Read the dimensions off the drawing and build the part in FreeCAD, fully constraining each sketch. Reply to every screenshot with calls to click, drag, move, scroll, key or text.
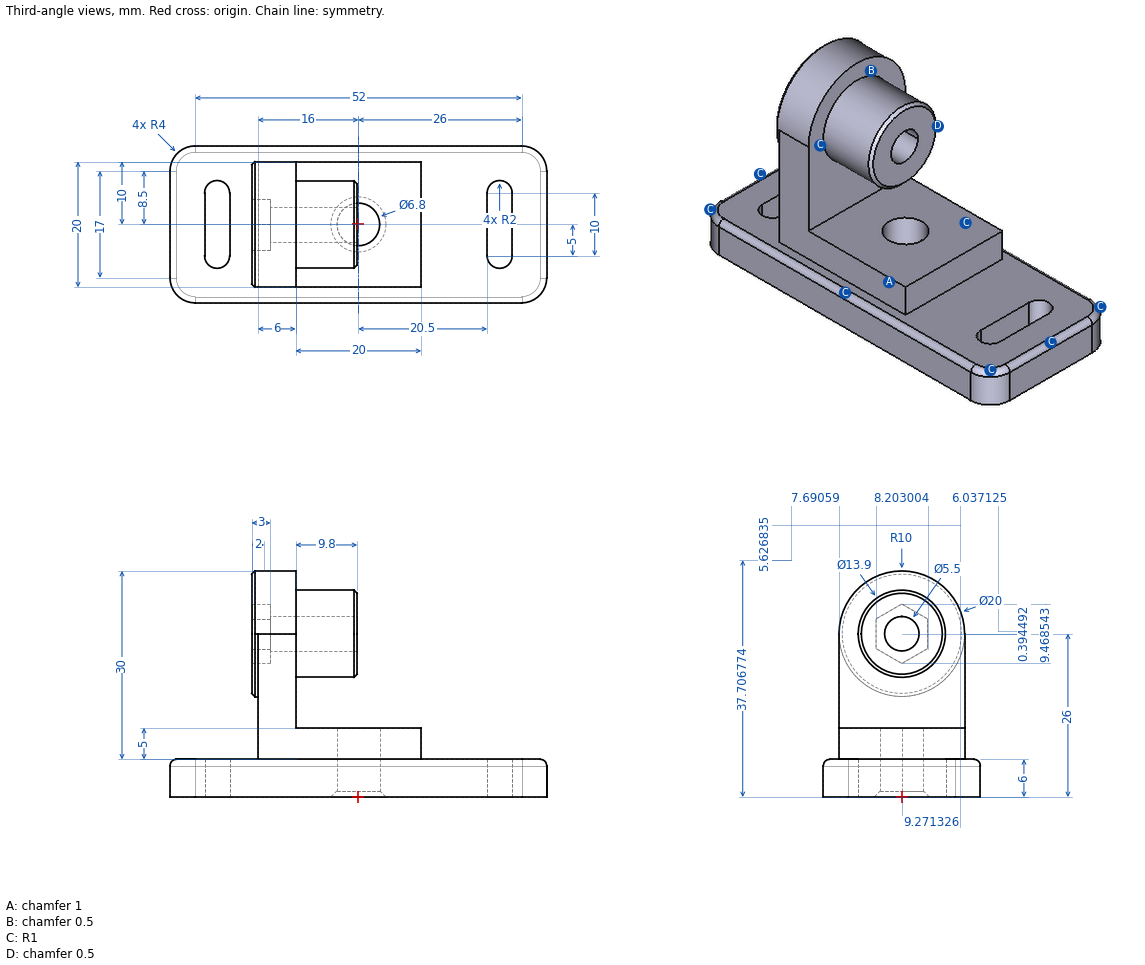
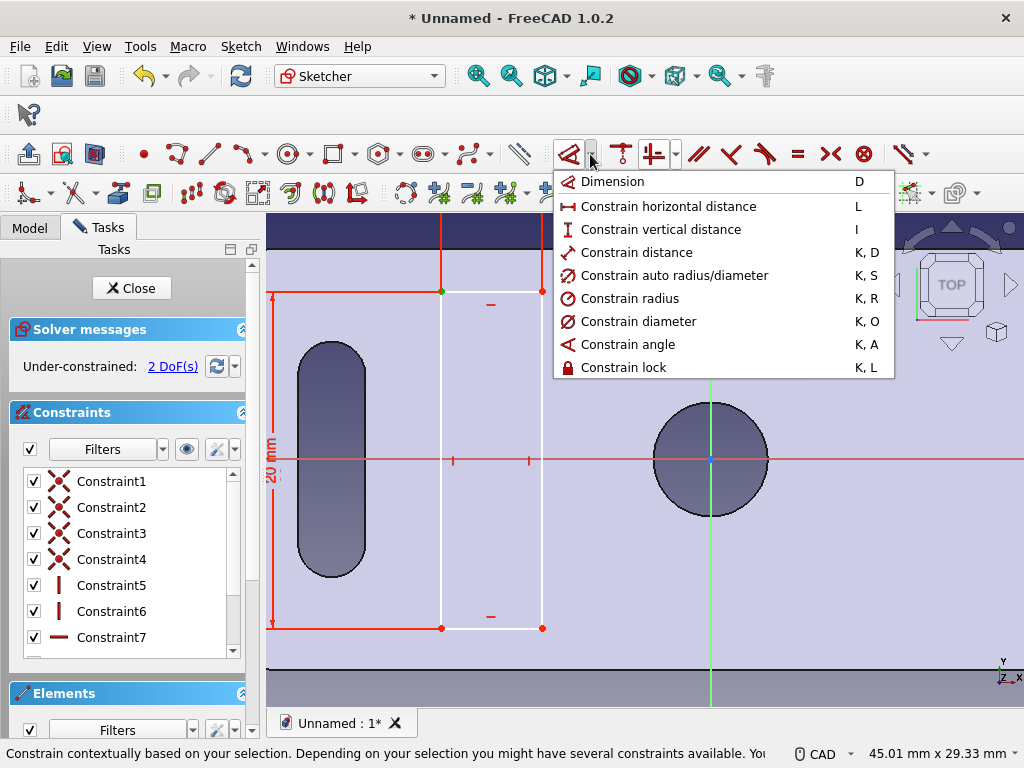
click(724, 206)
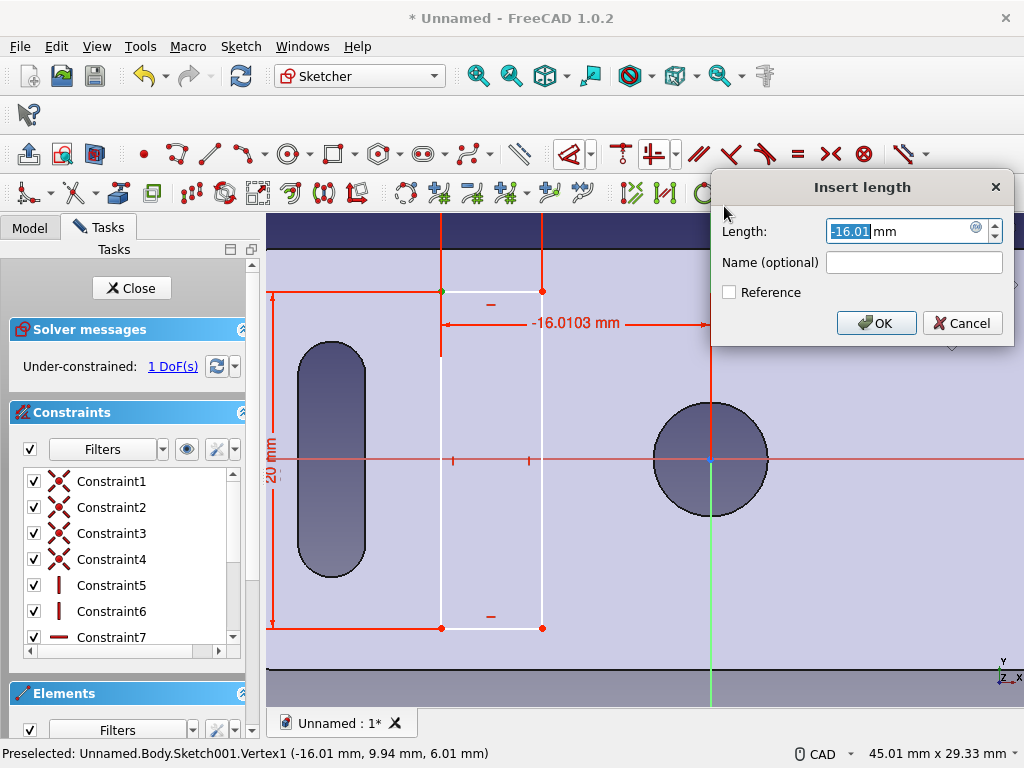
text(-16)
key(Return)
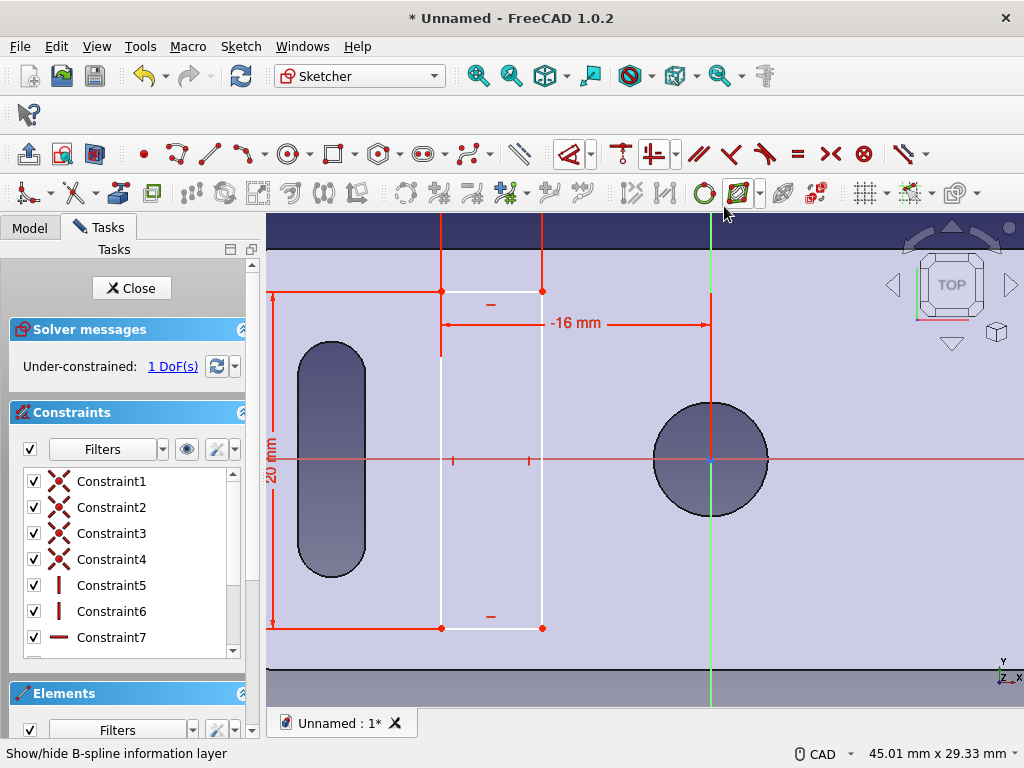
click(441, 292)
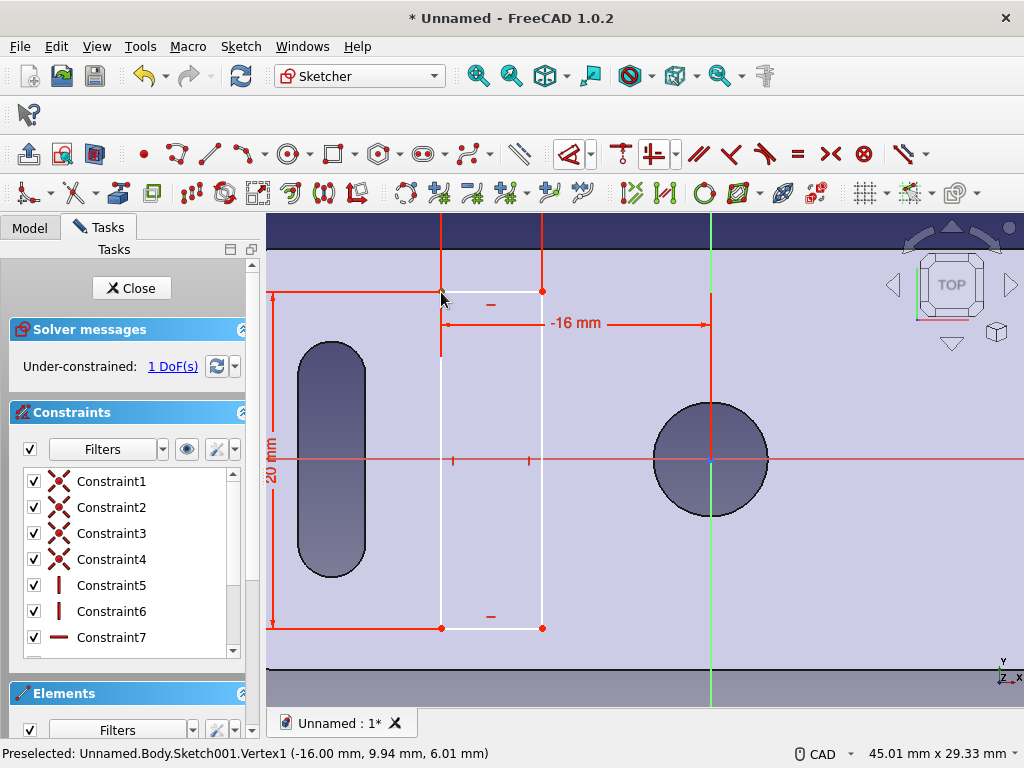
key(i)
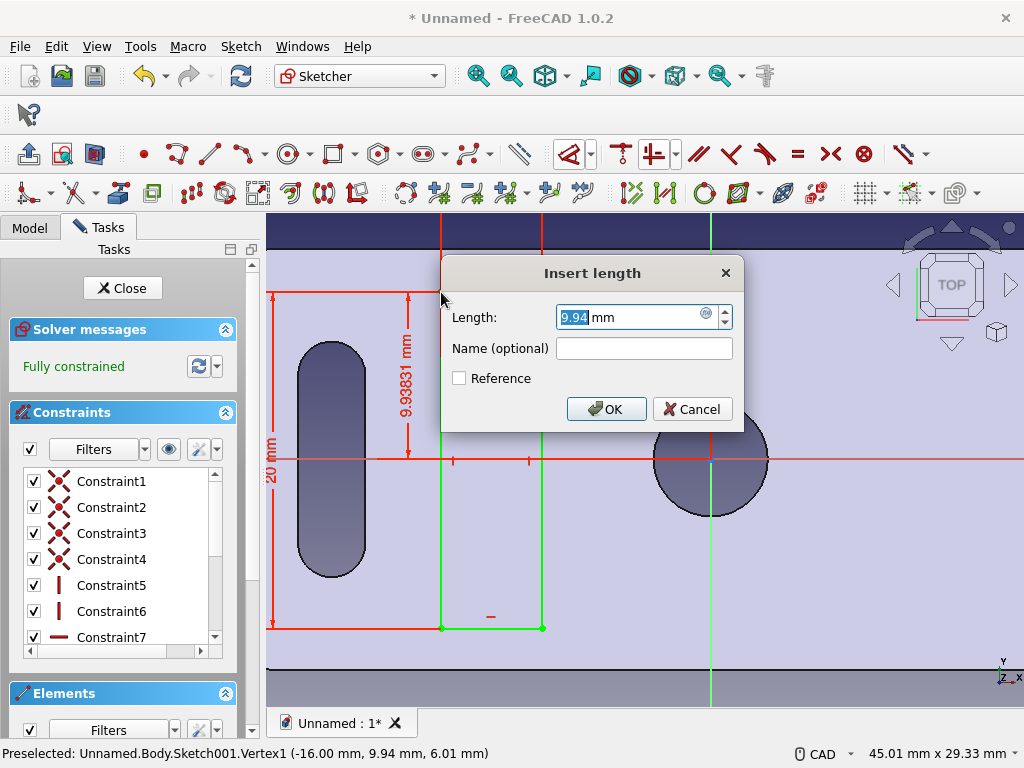
text(10)
key(Return)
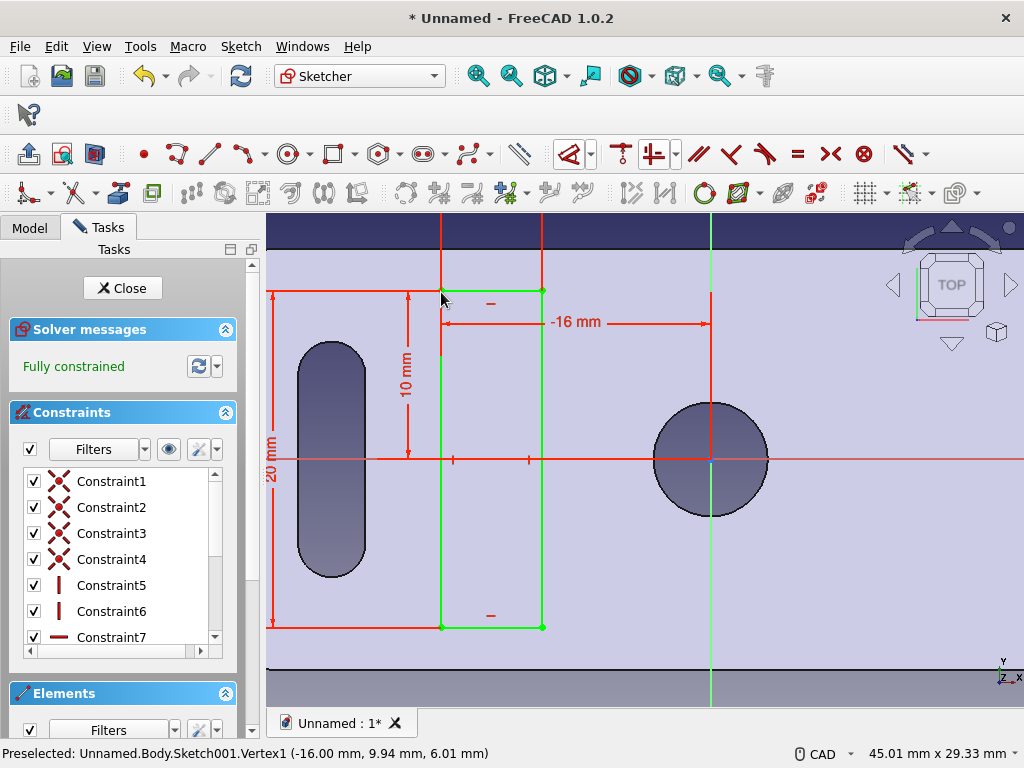
click(123, 288)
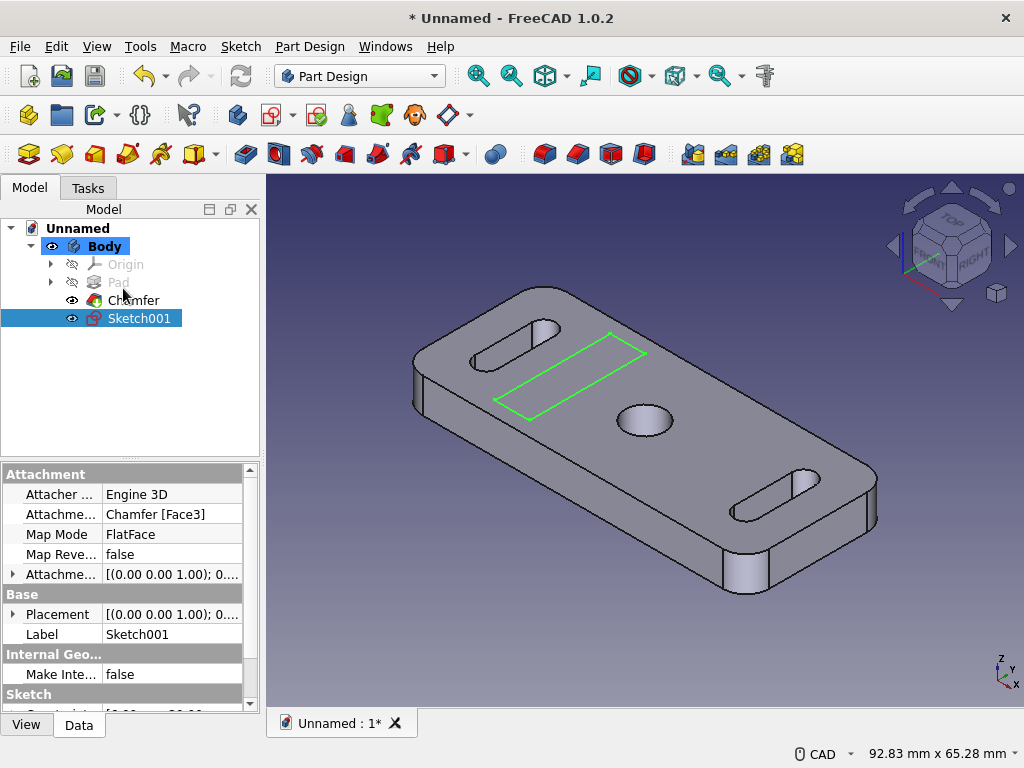
click(29, 154)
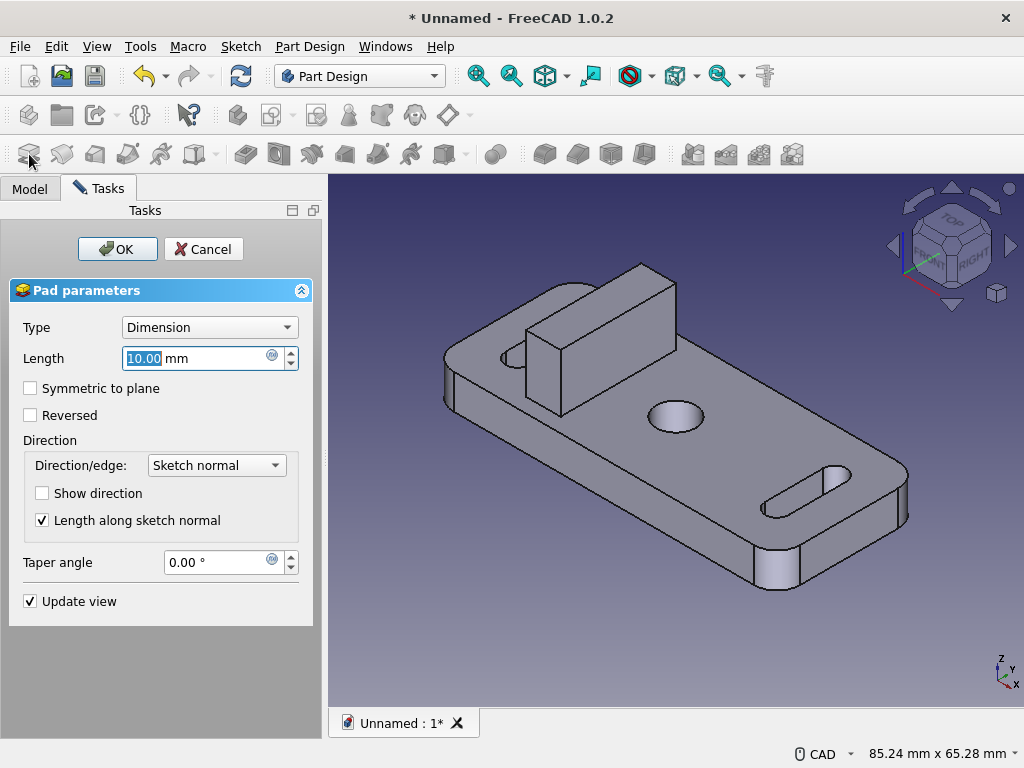
text(30)
key(Tab)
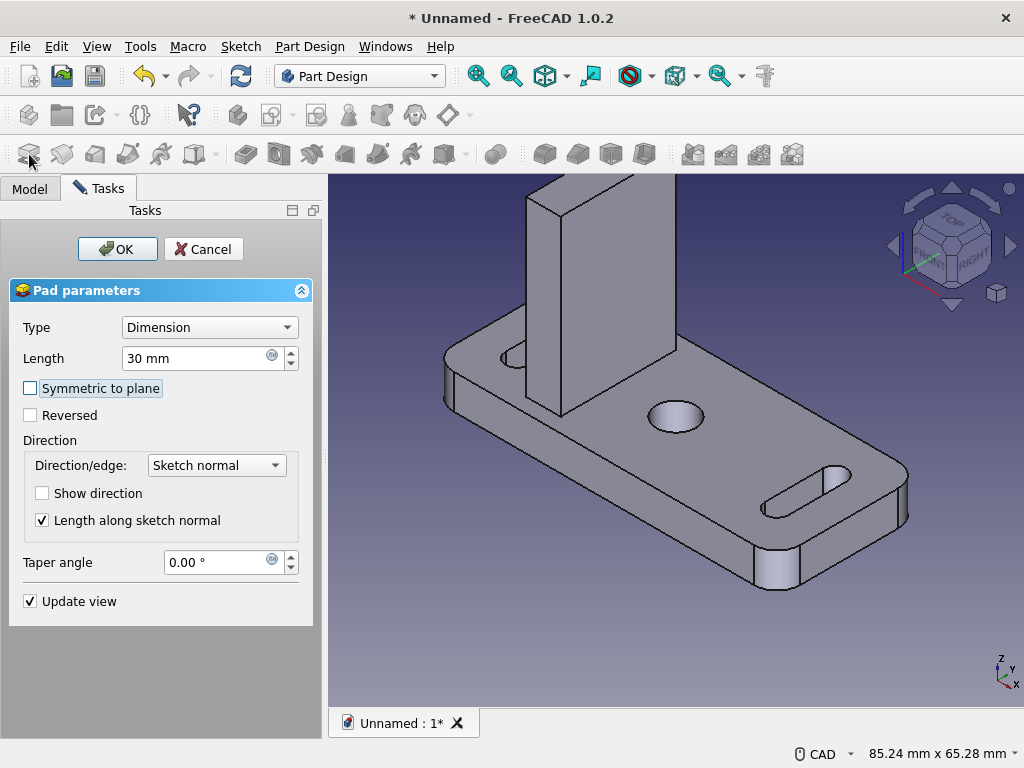
click(118, 249)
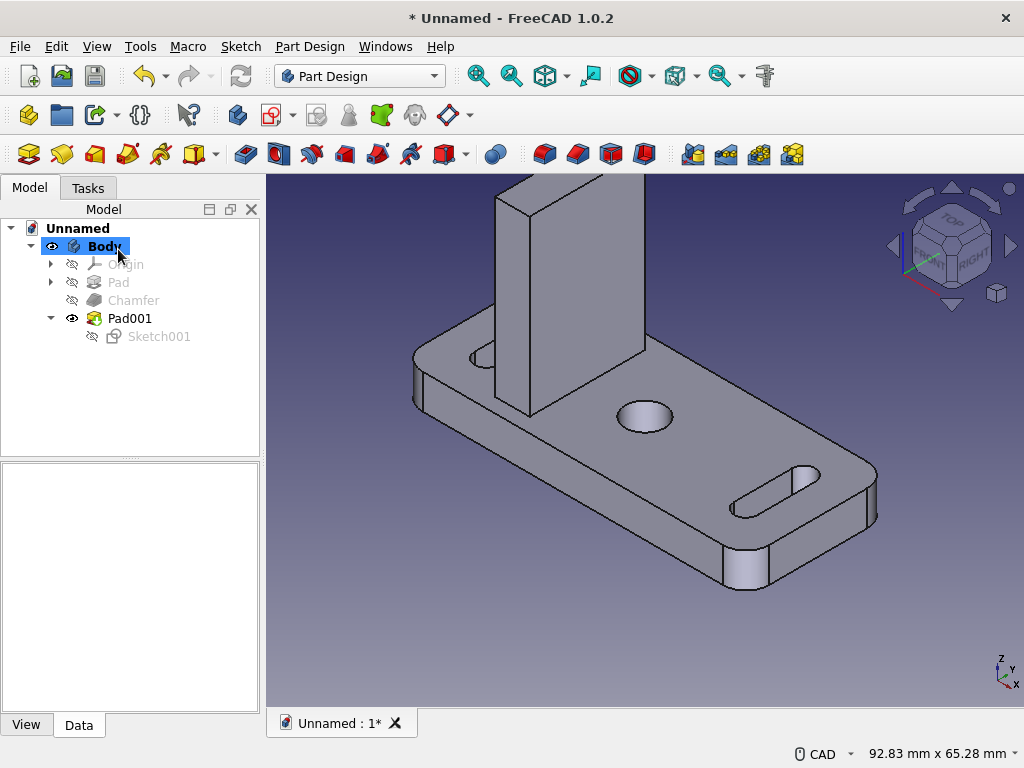
click(479, 76)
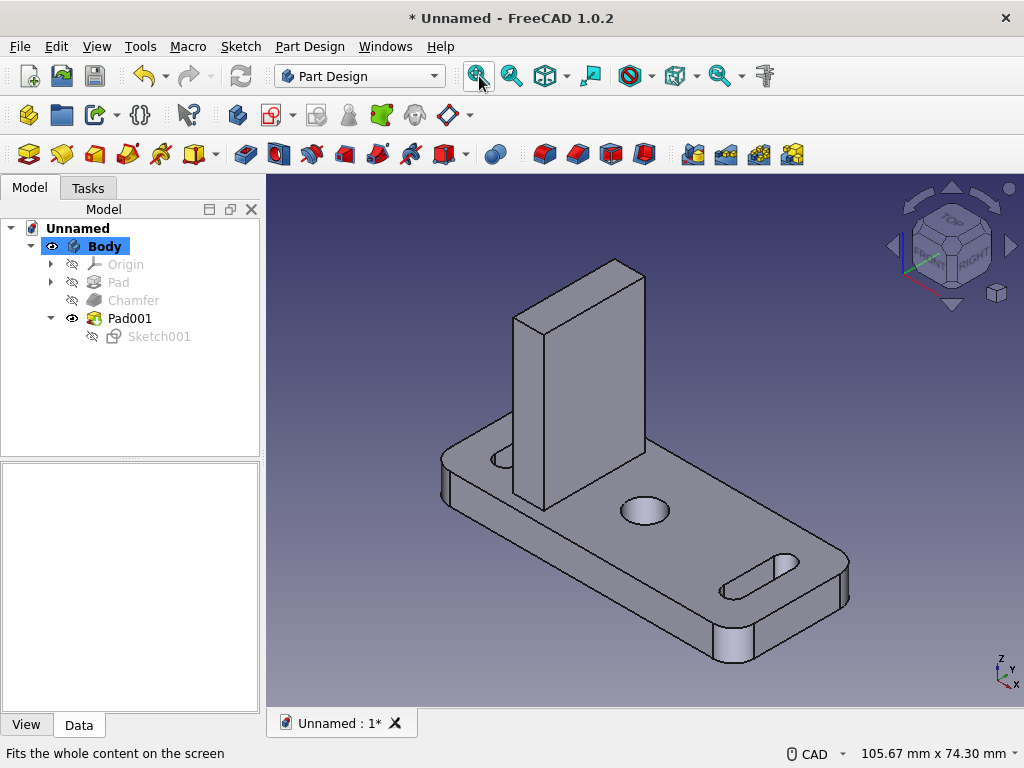
key(6)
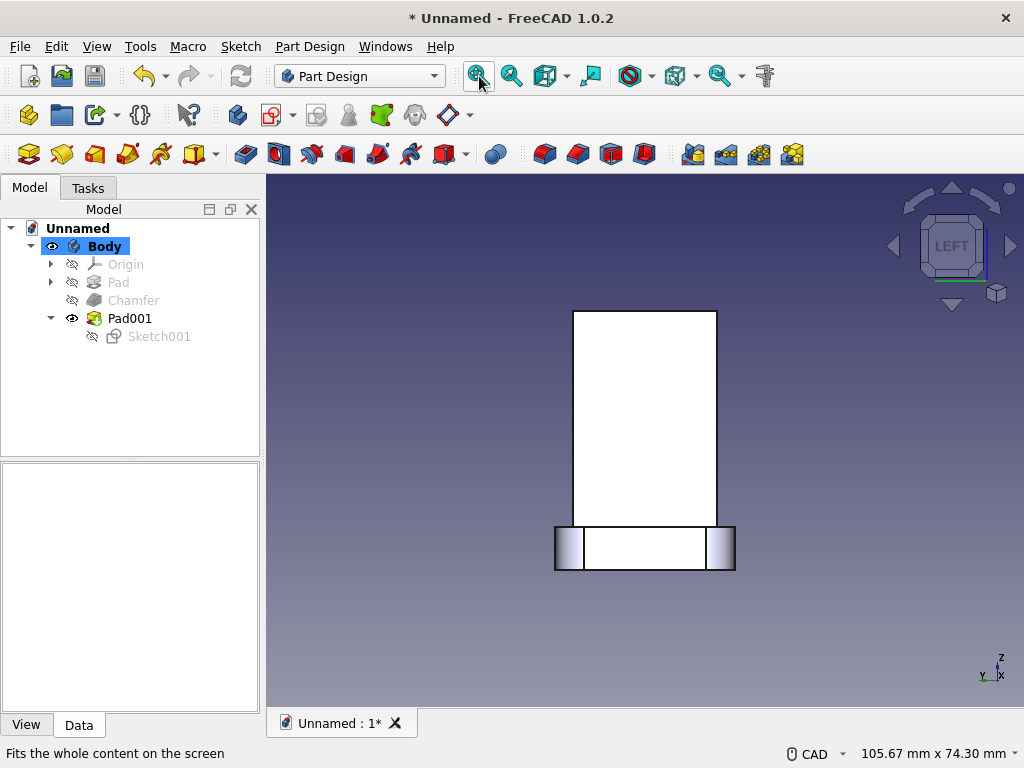
click(645, 387)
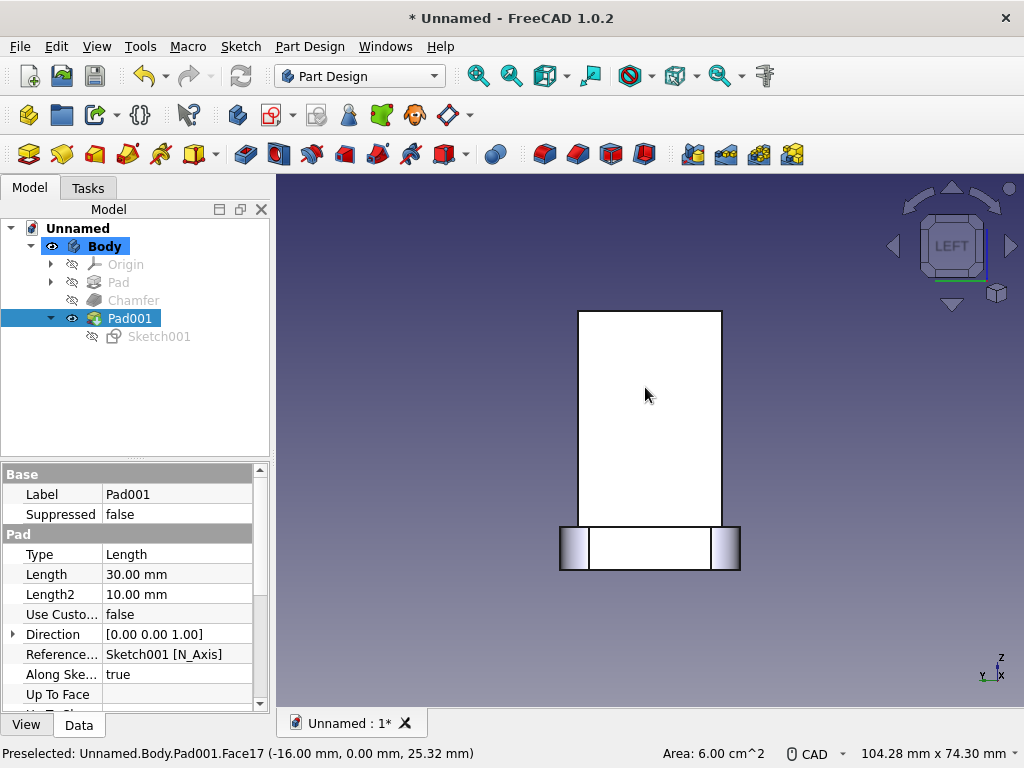
click(270, 116)